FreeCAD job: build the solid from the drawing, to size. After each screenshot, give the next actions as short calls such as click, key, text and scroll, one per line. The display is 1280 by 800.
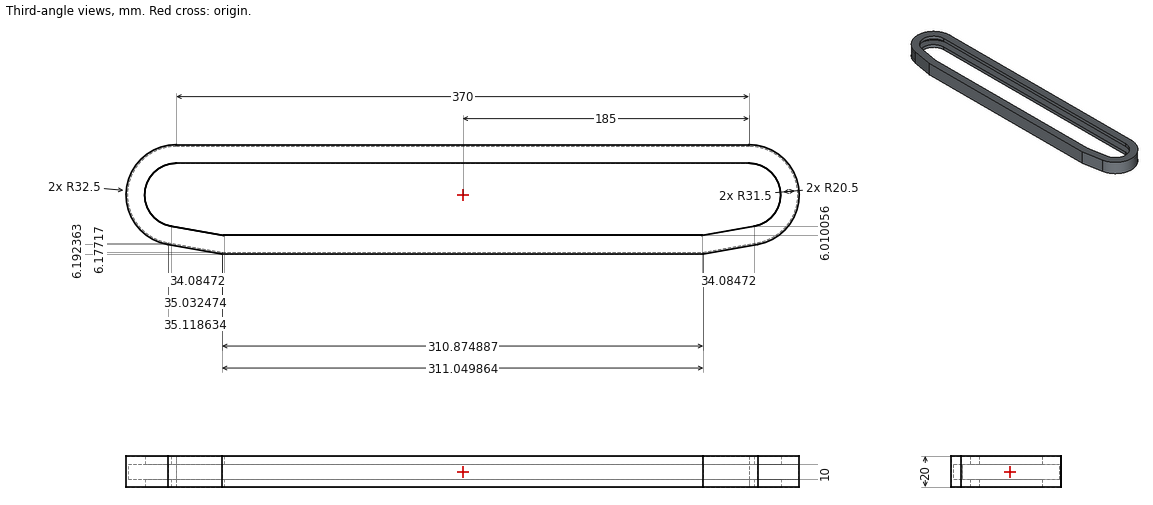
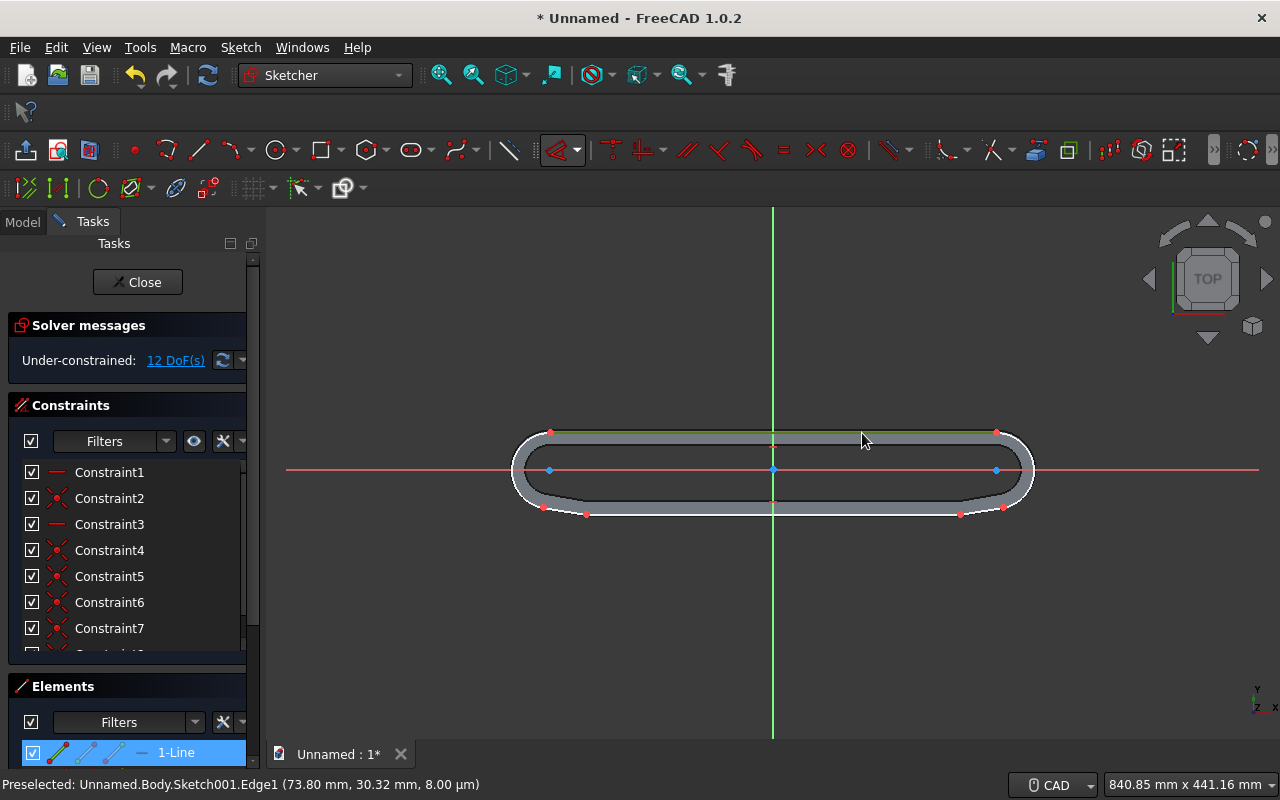
click(521, 447)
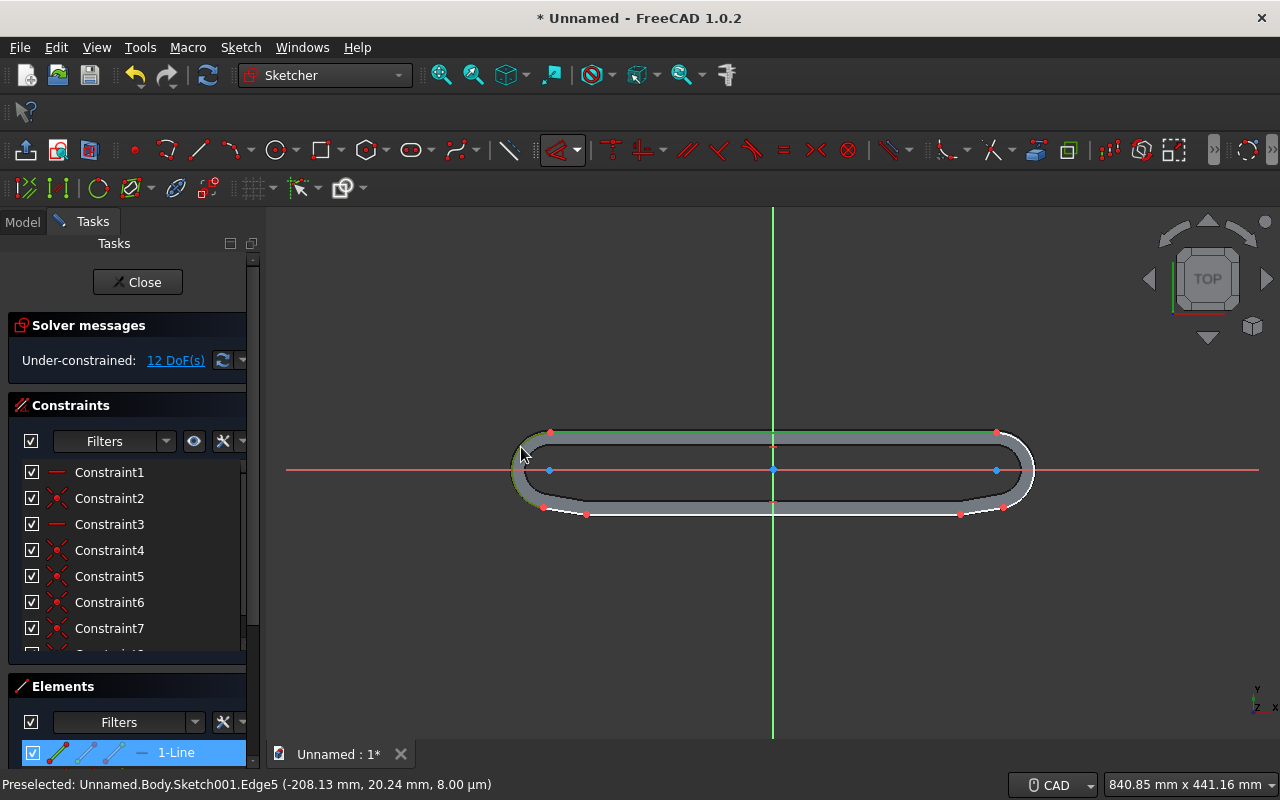
key(t)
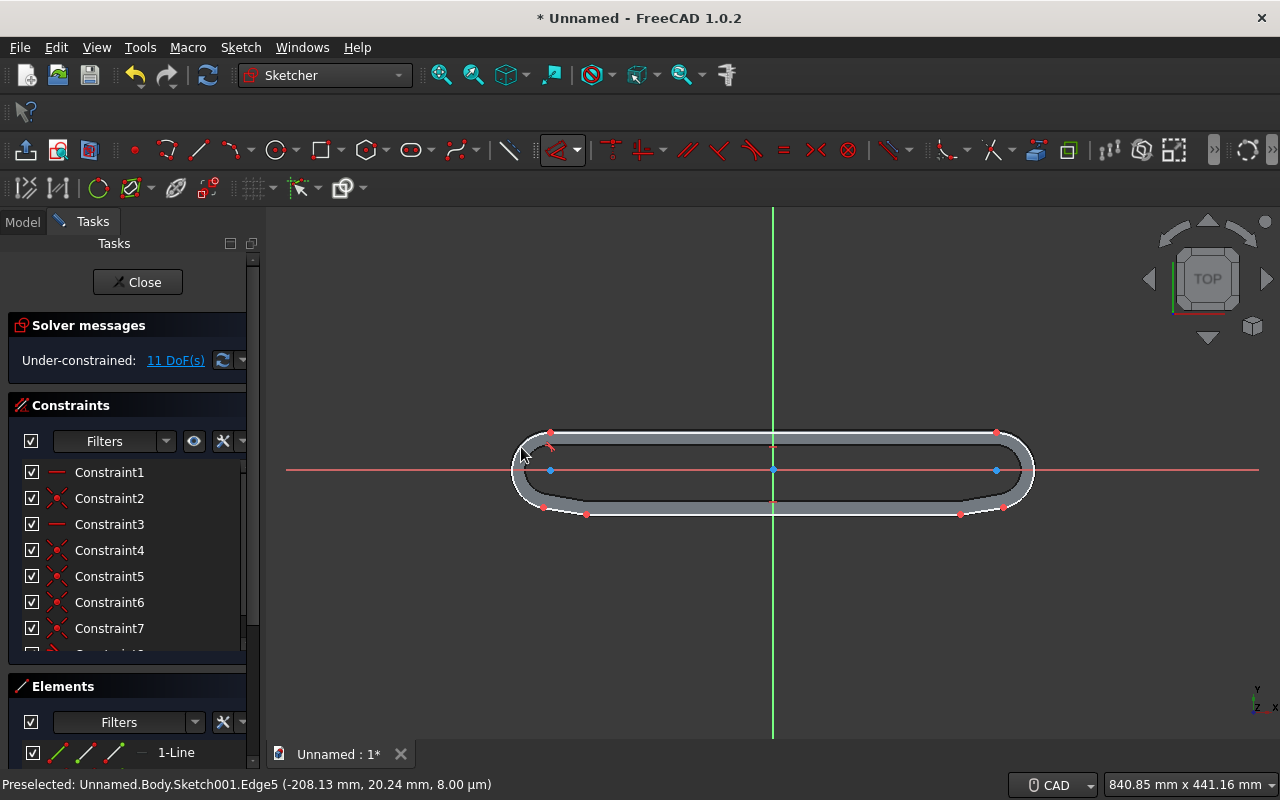
click(862, 433)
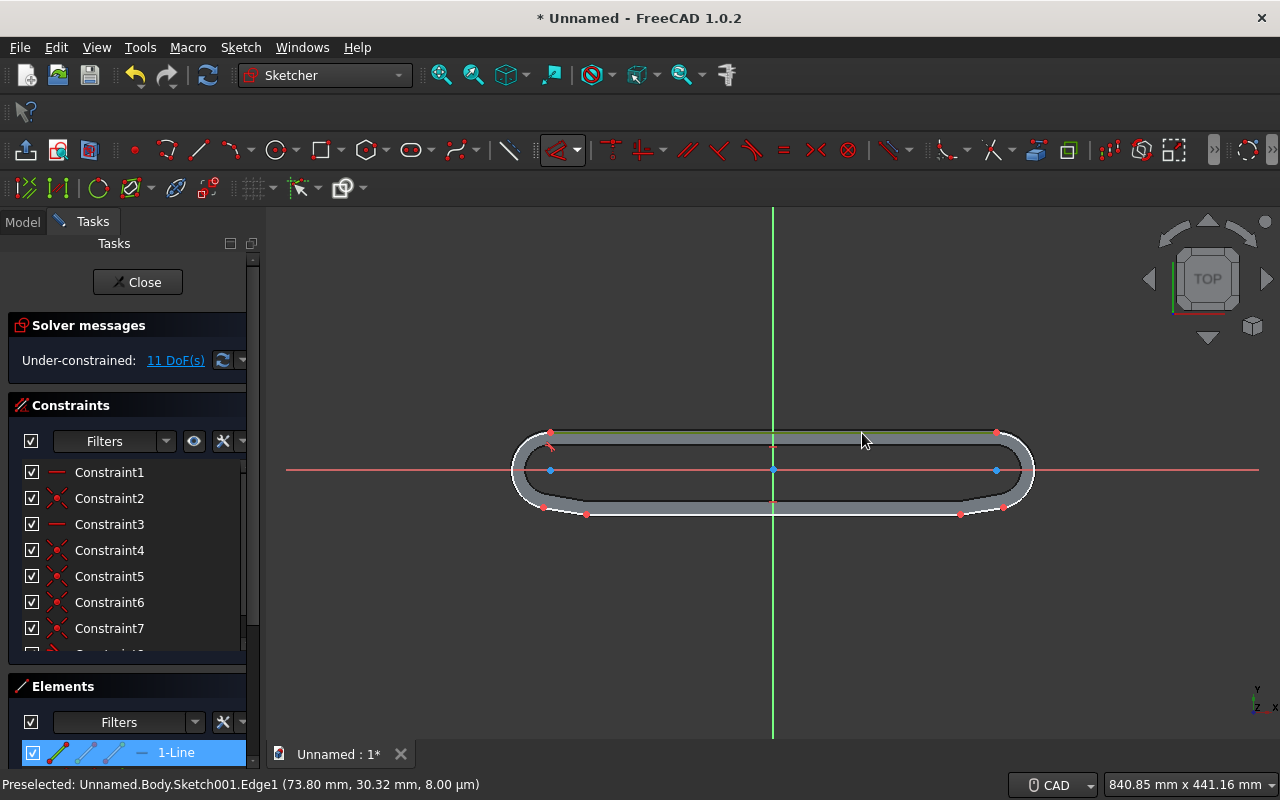
click(1029, 489)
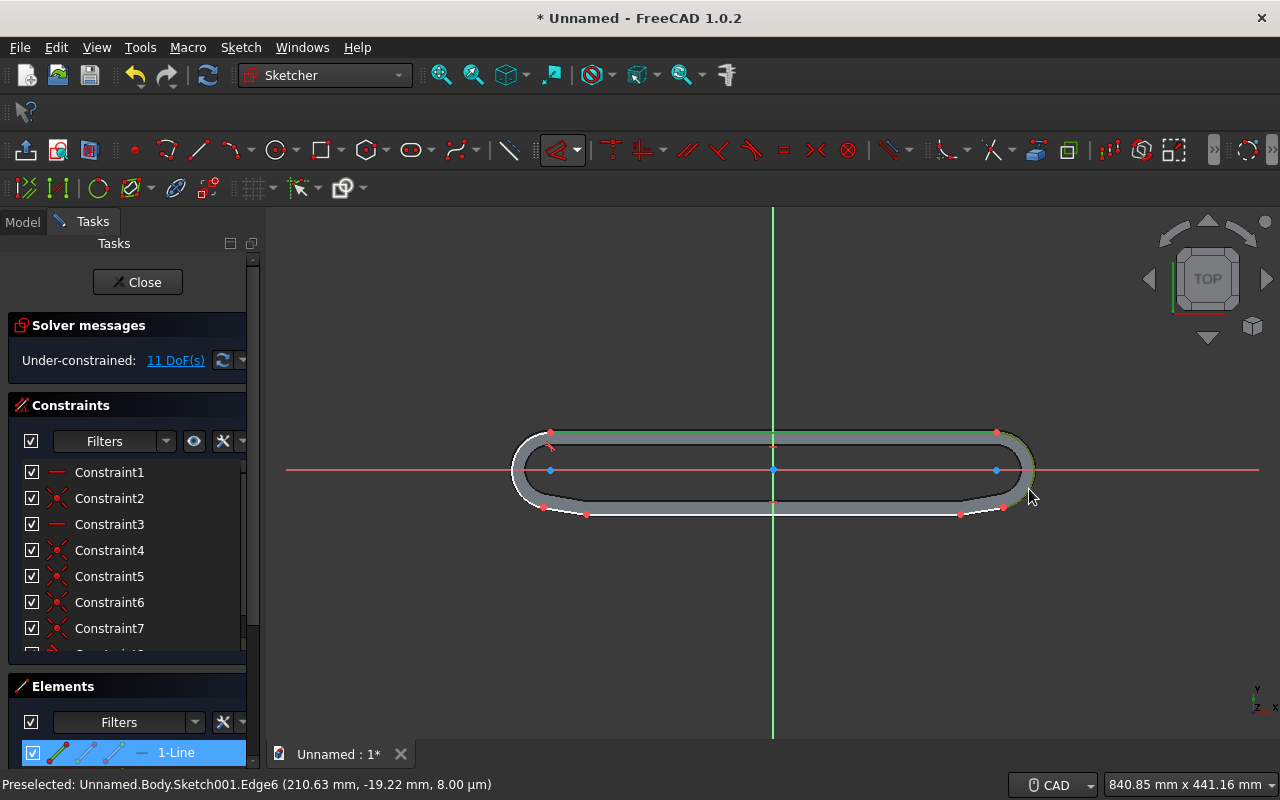
key(t)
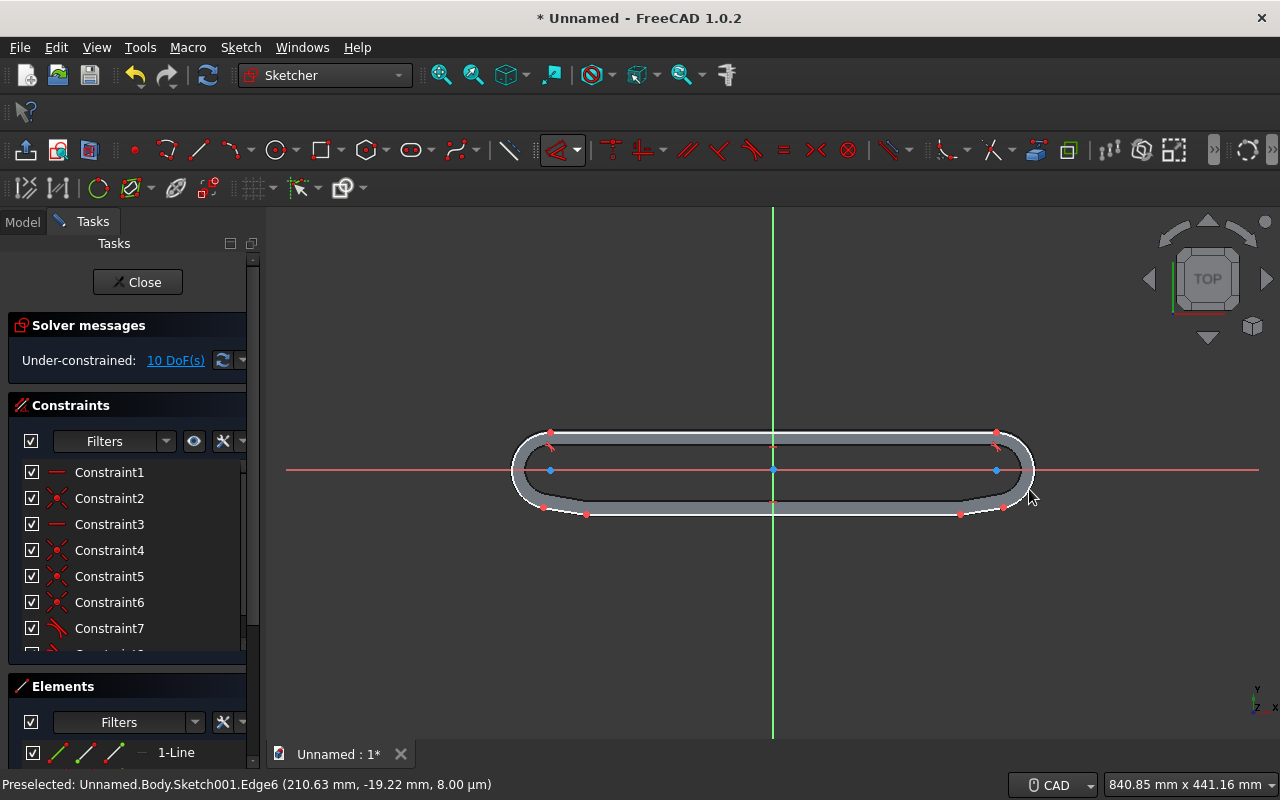
click(556, 510)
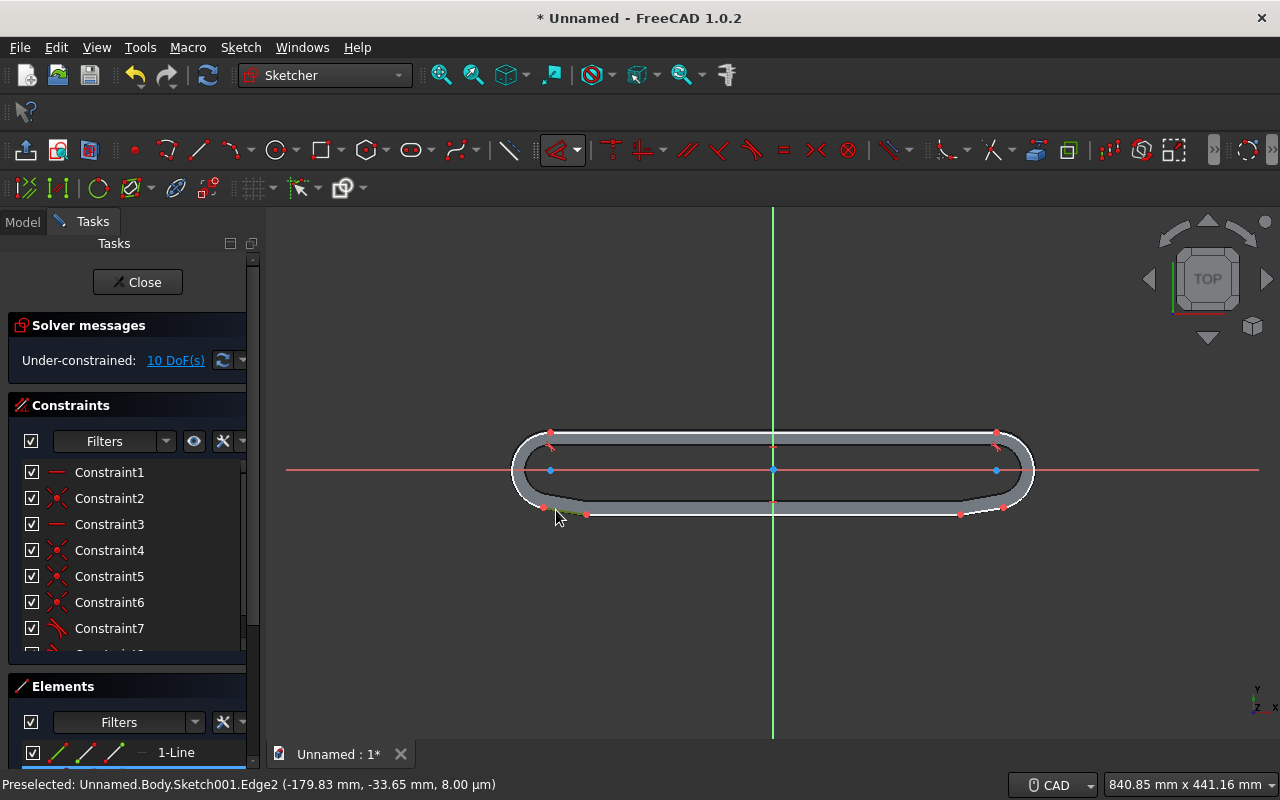
click(521, 447)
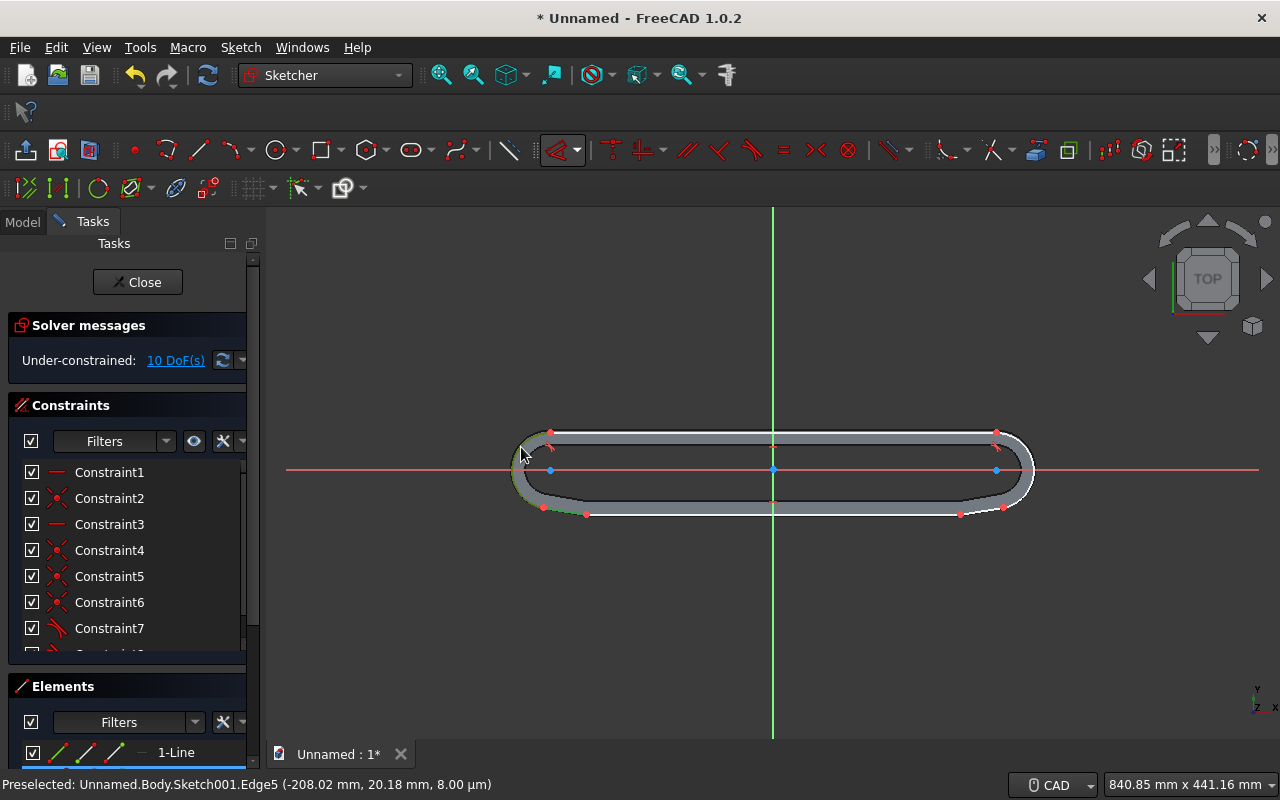
click(752, 150)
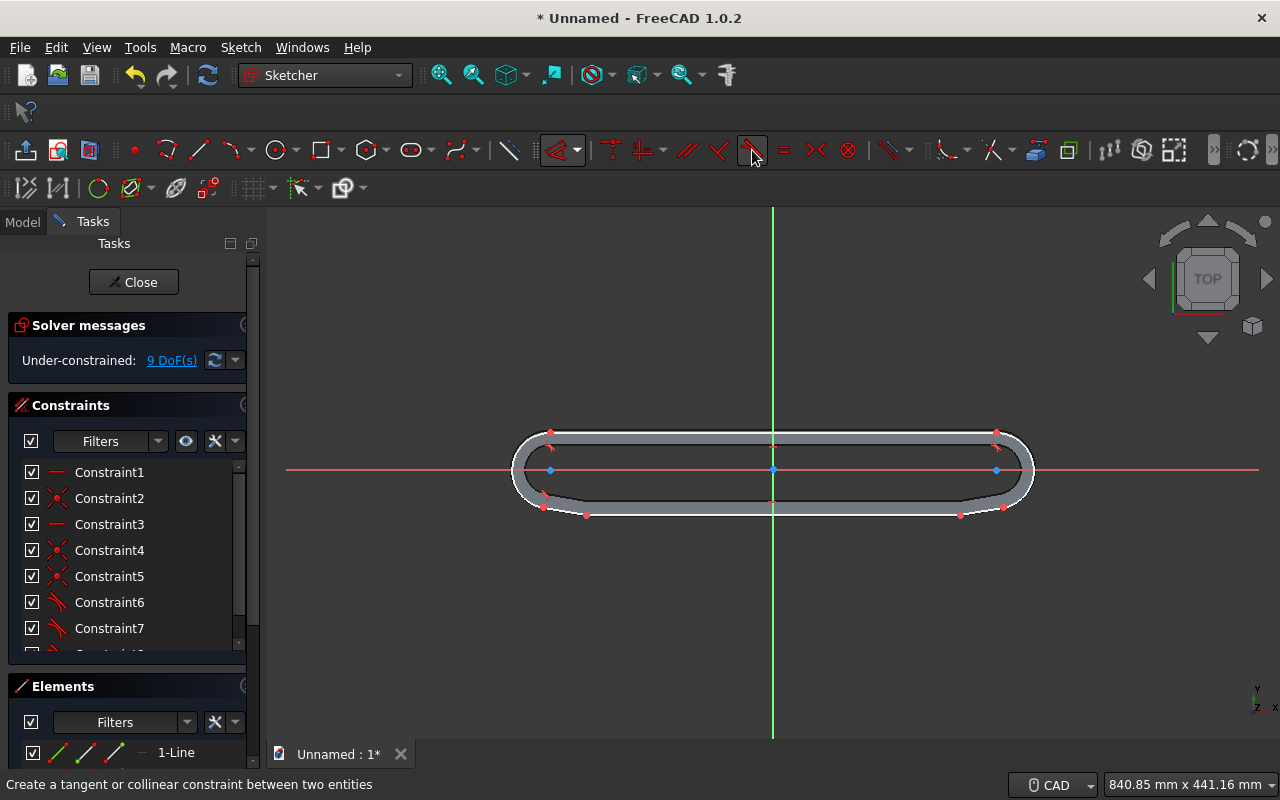
click(973, 513)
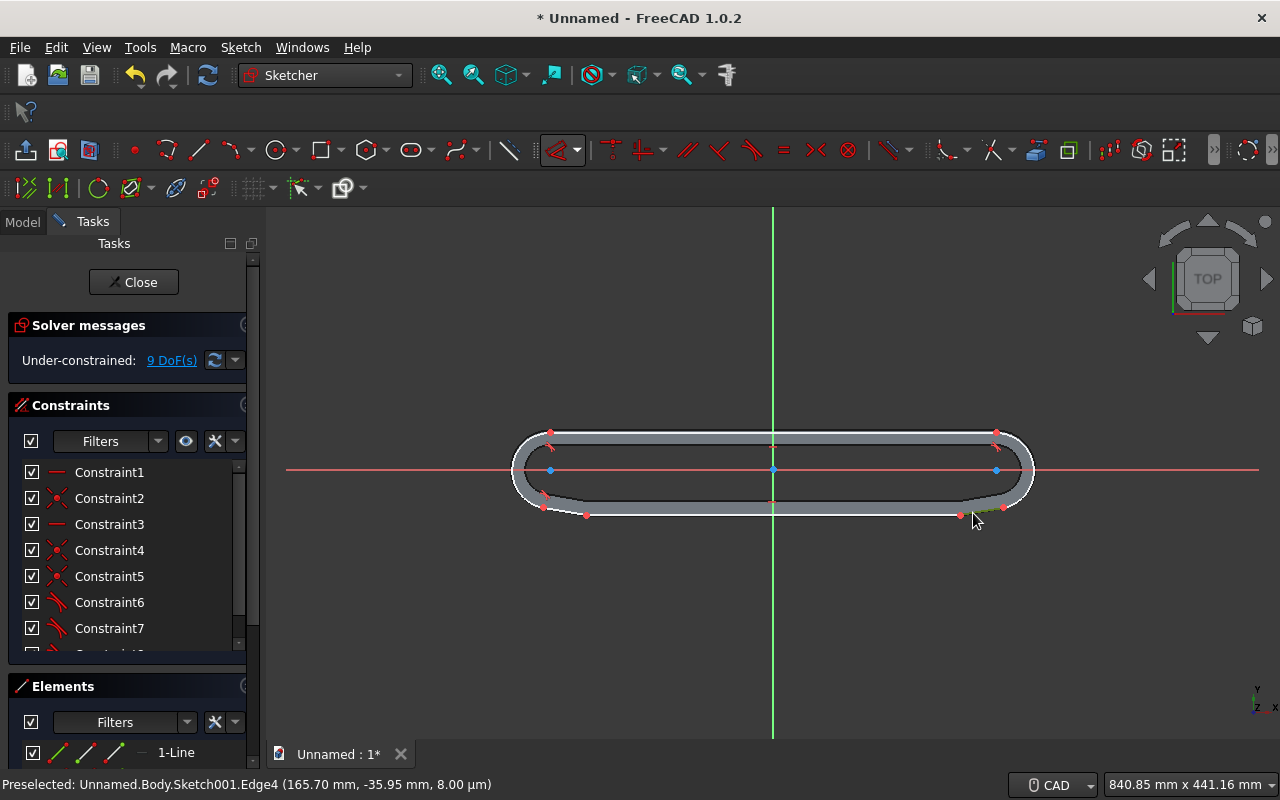
click(1029, 489)